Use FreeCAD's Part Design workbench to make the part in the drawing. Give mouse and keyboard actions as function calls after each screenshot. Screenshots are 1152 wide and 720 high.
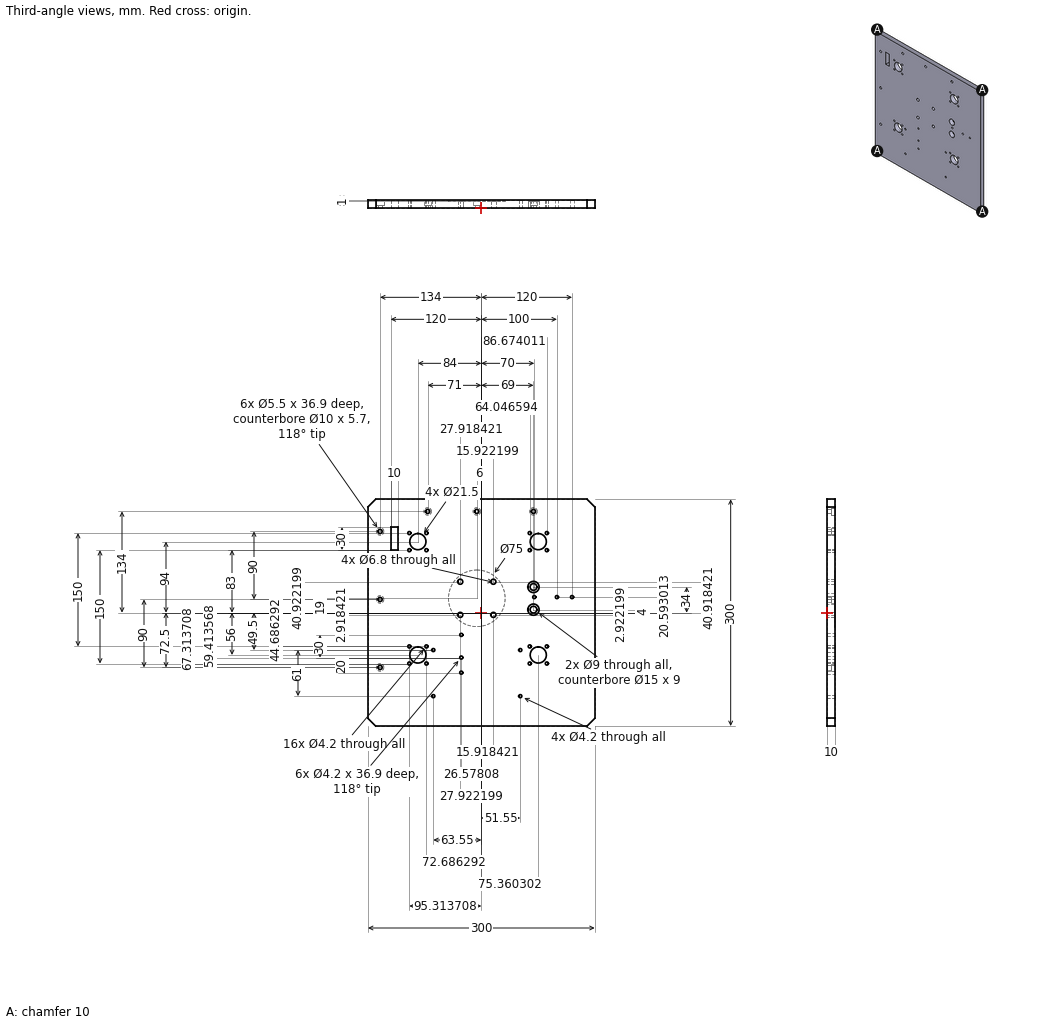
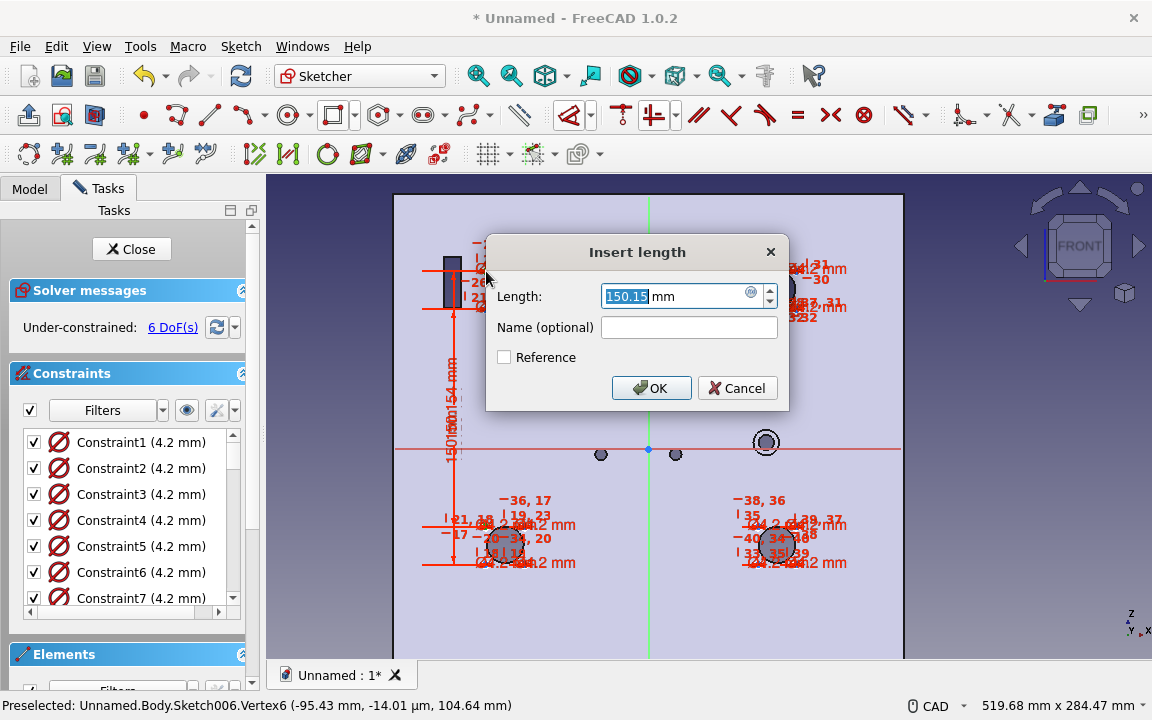
text(150)
key(Return)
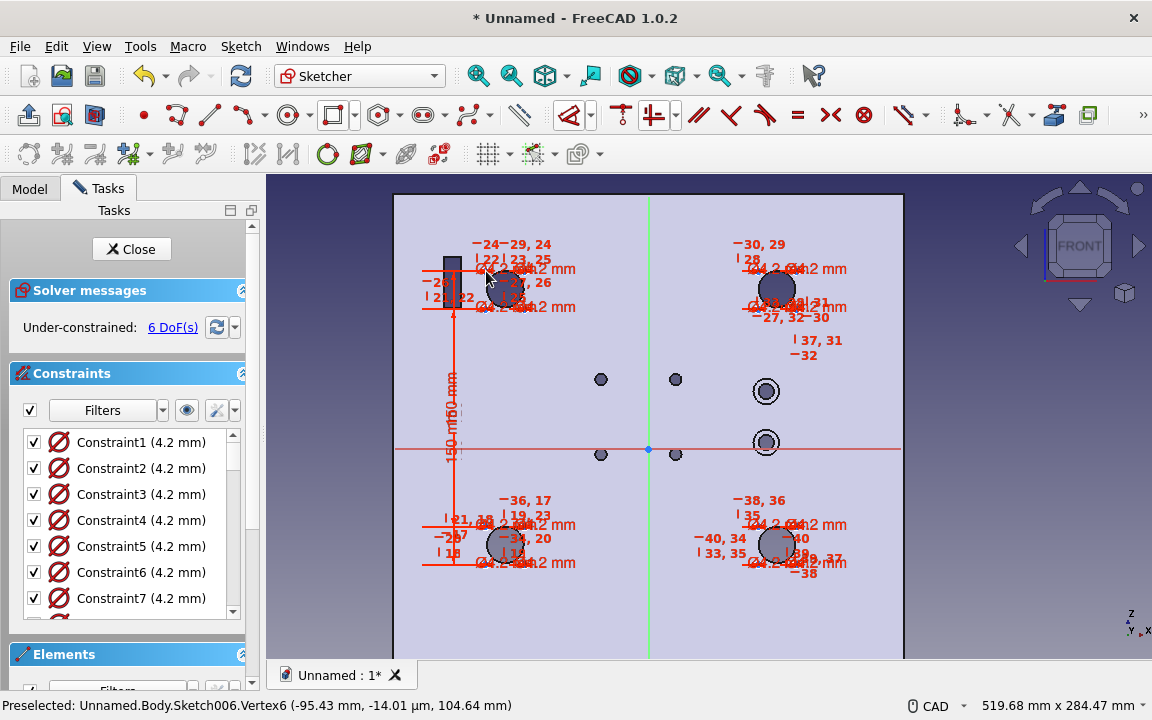
click(525, 527)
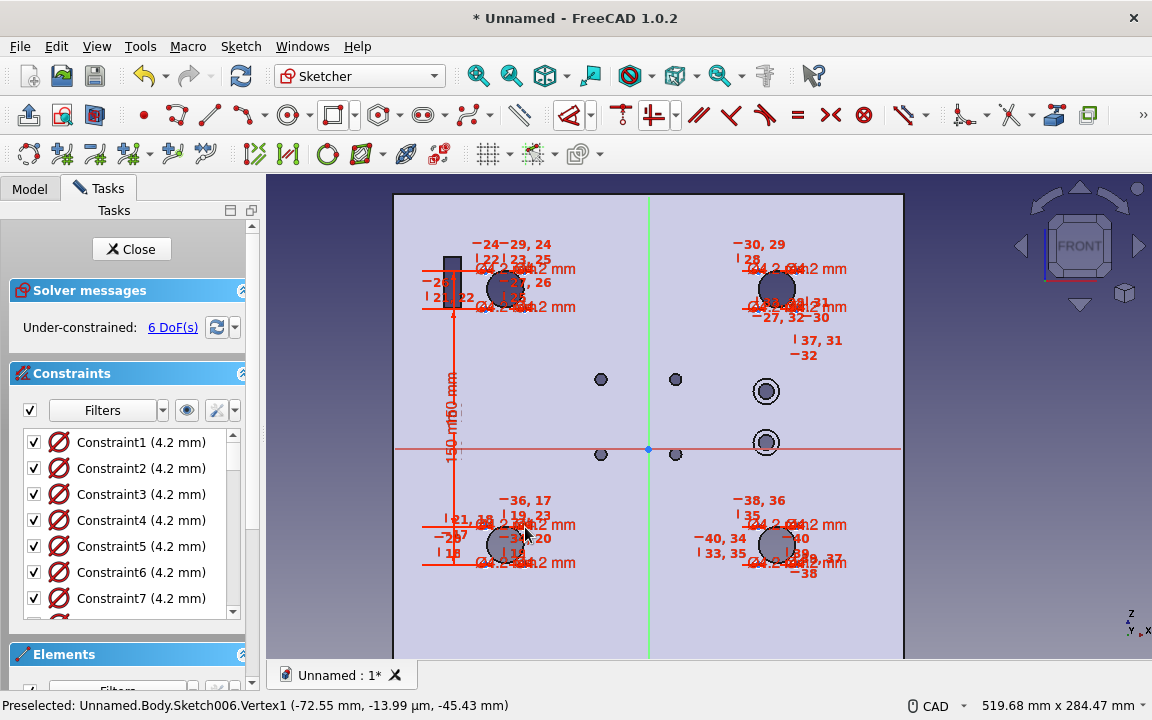
key(l)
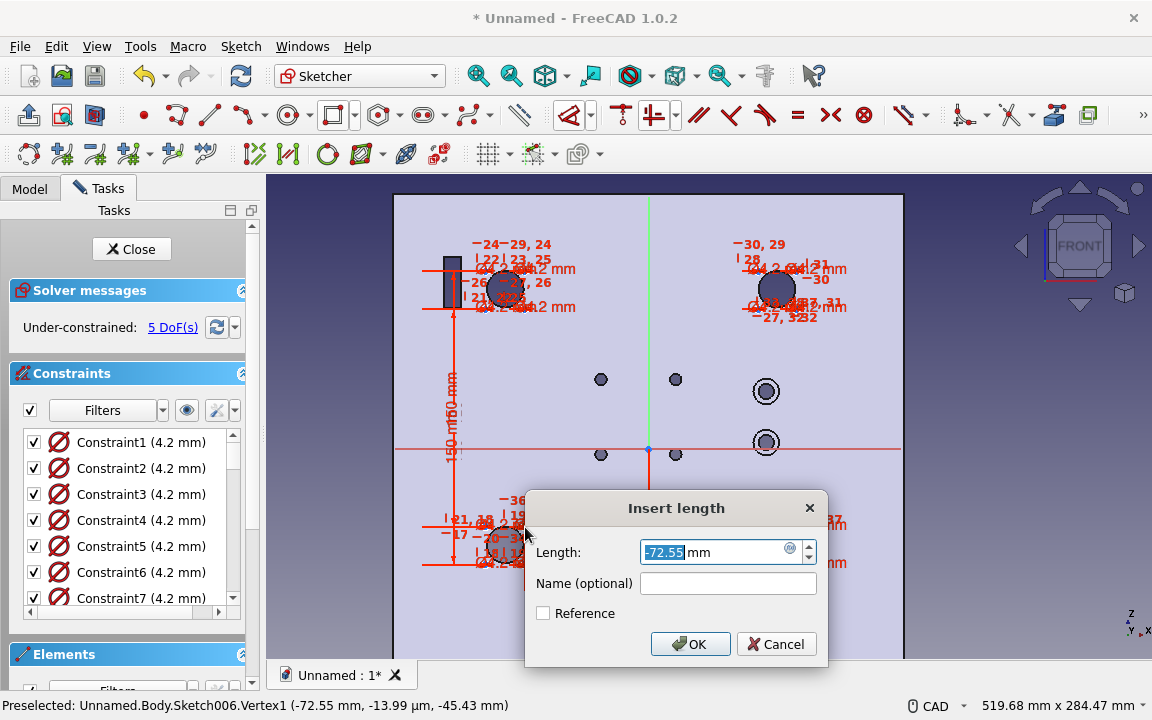
text(-72.686292)
key(Return)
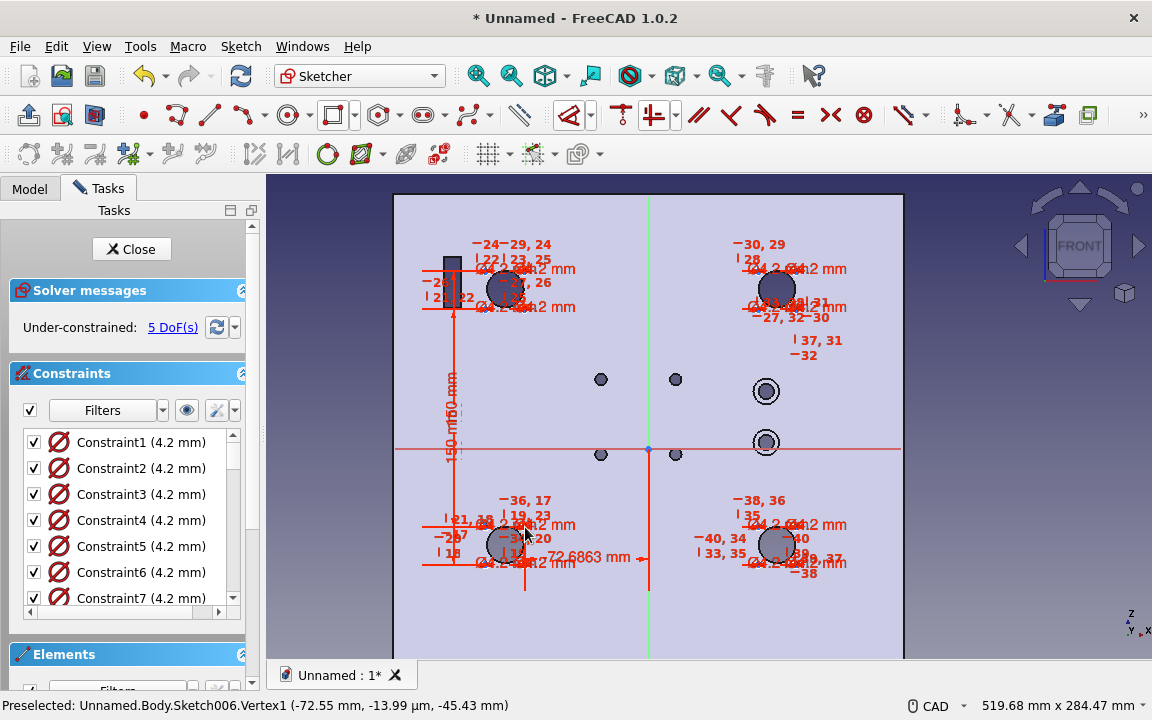
click(525, 527)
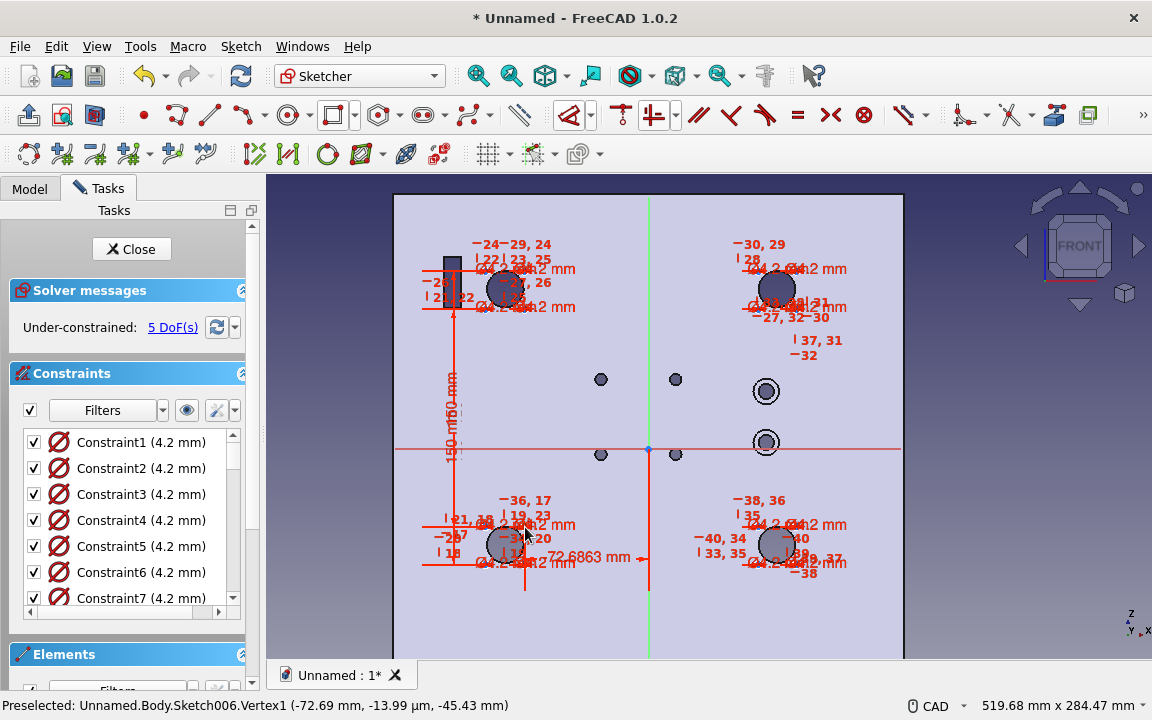
key(i)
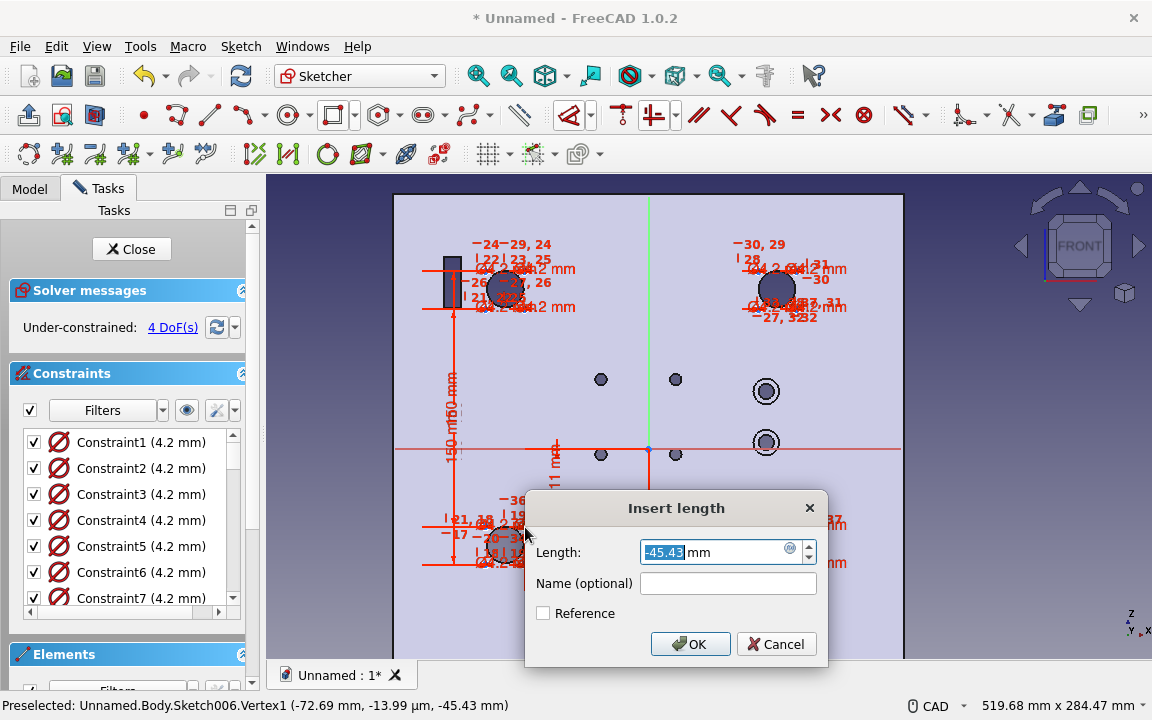
text(-44.686292)
key(Return)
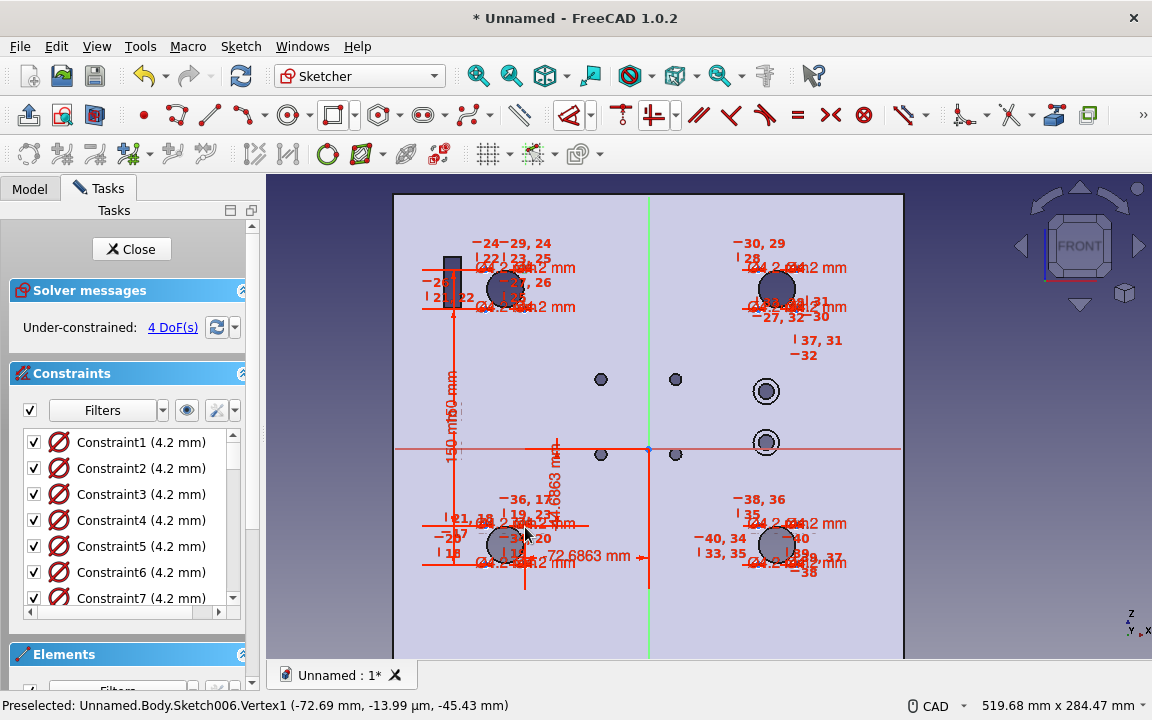
click(486, 526)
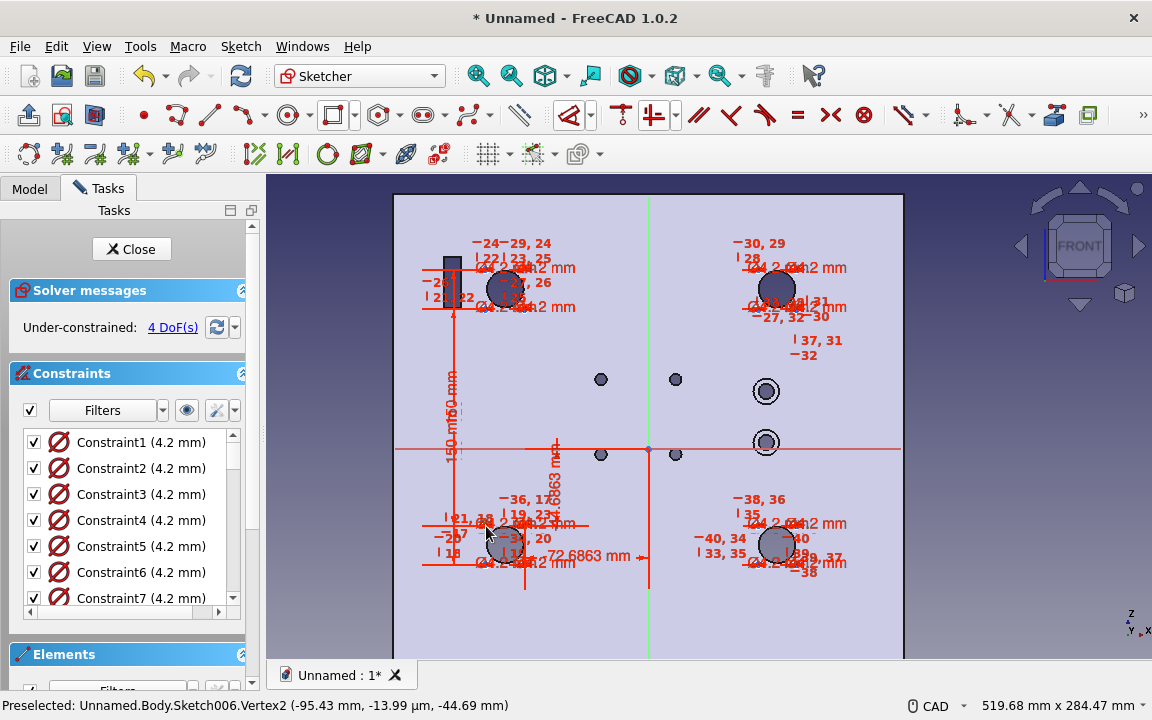
key(l)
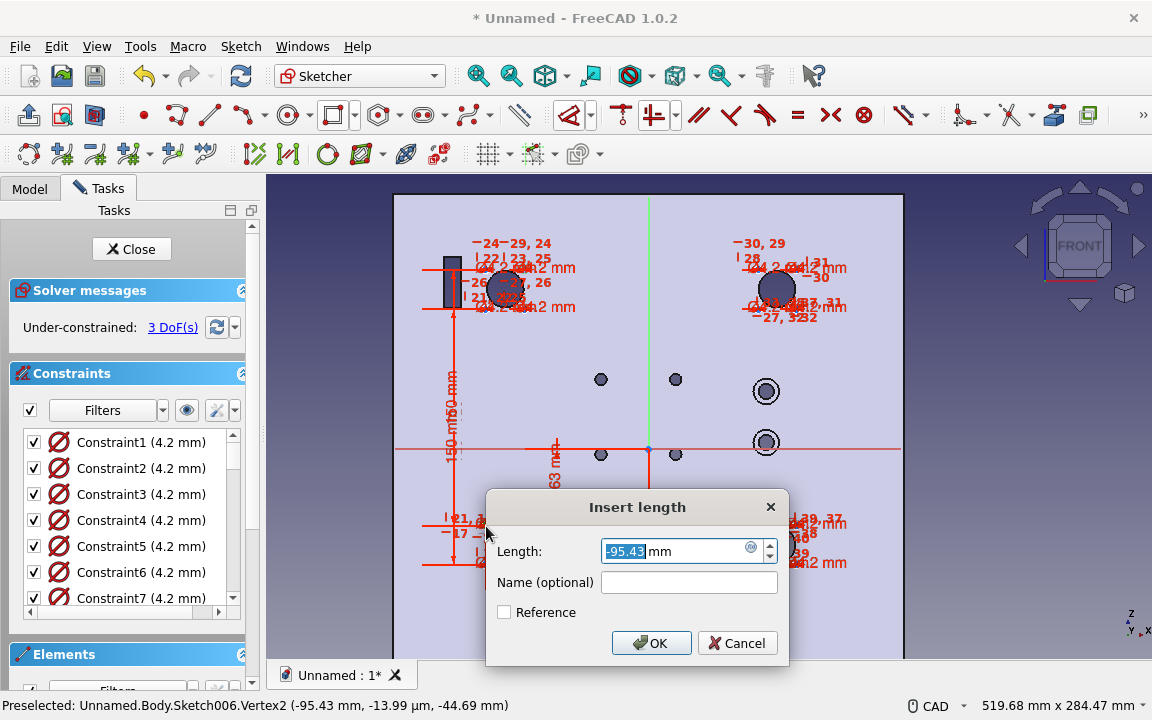
text(-95.313708)
key(Return)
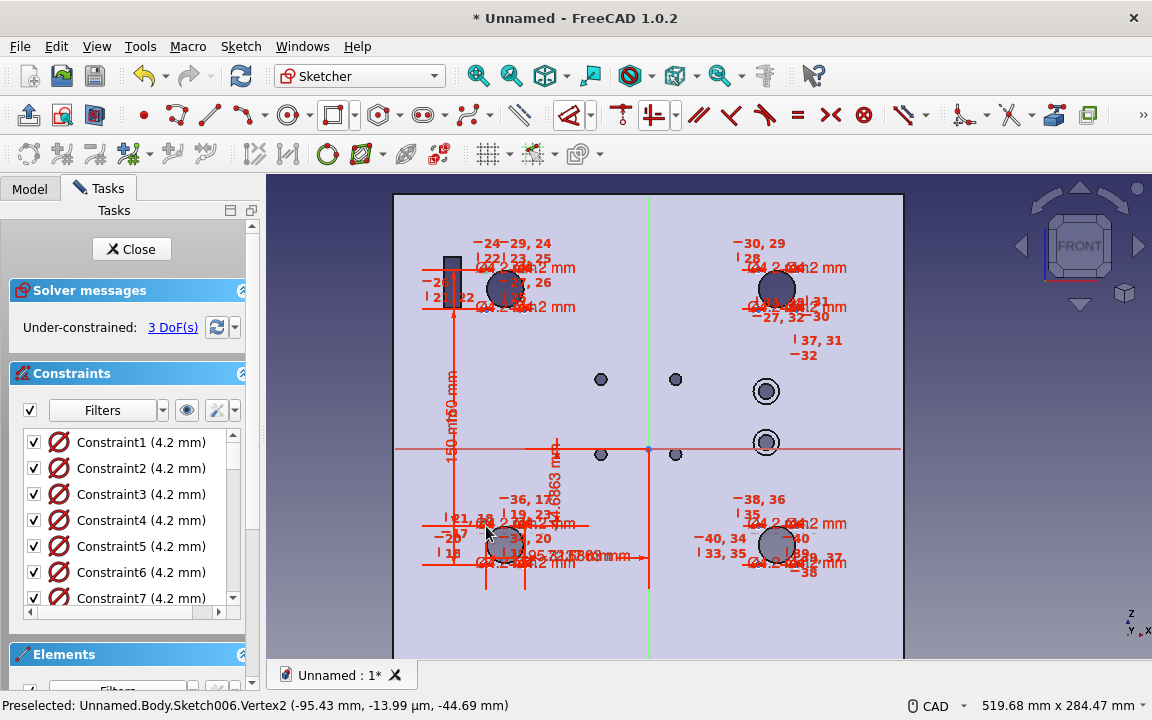
click(486, 565)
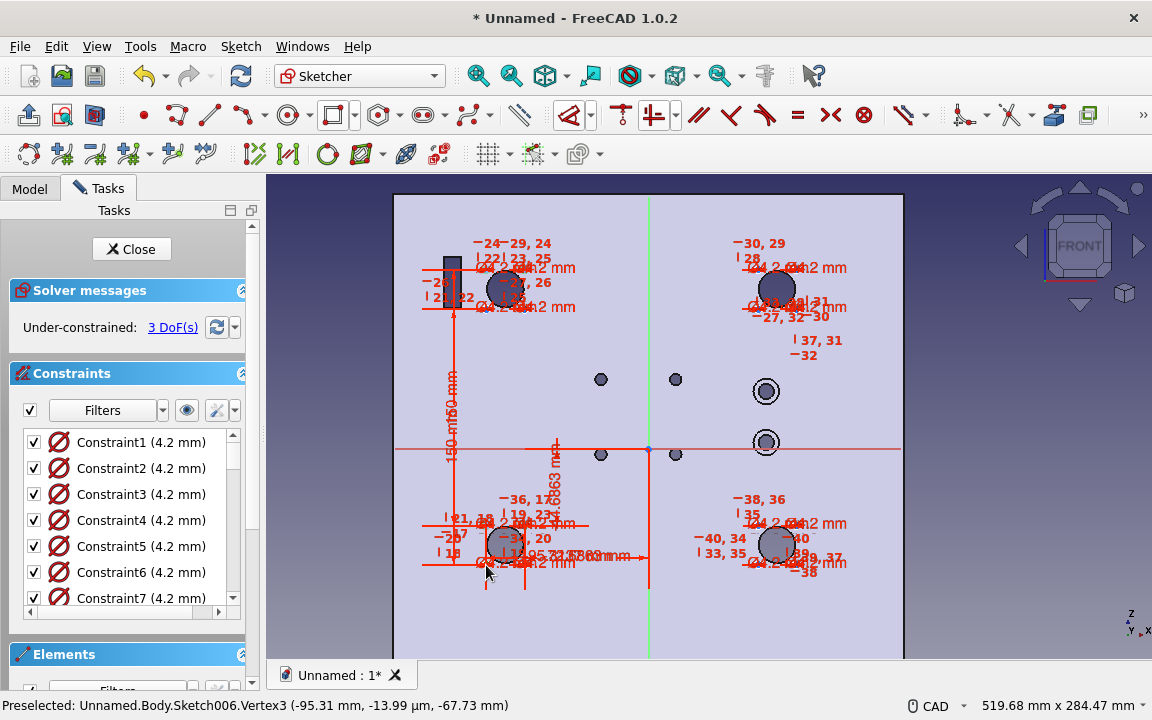
key(i)